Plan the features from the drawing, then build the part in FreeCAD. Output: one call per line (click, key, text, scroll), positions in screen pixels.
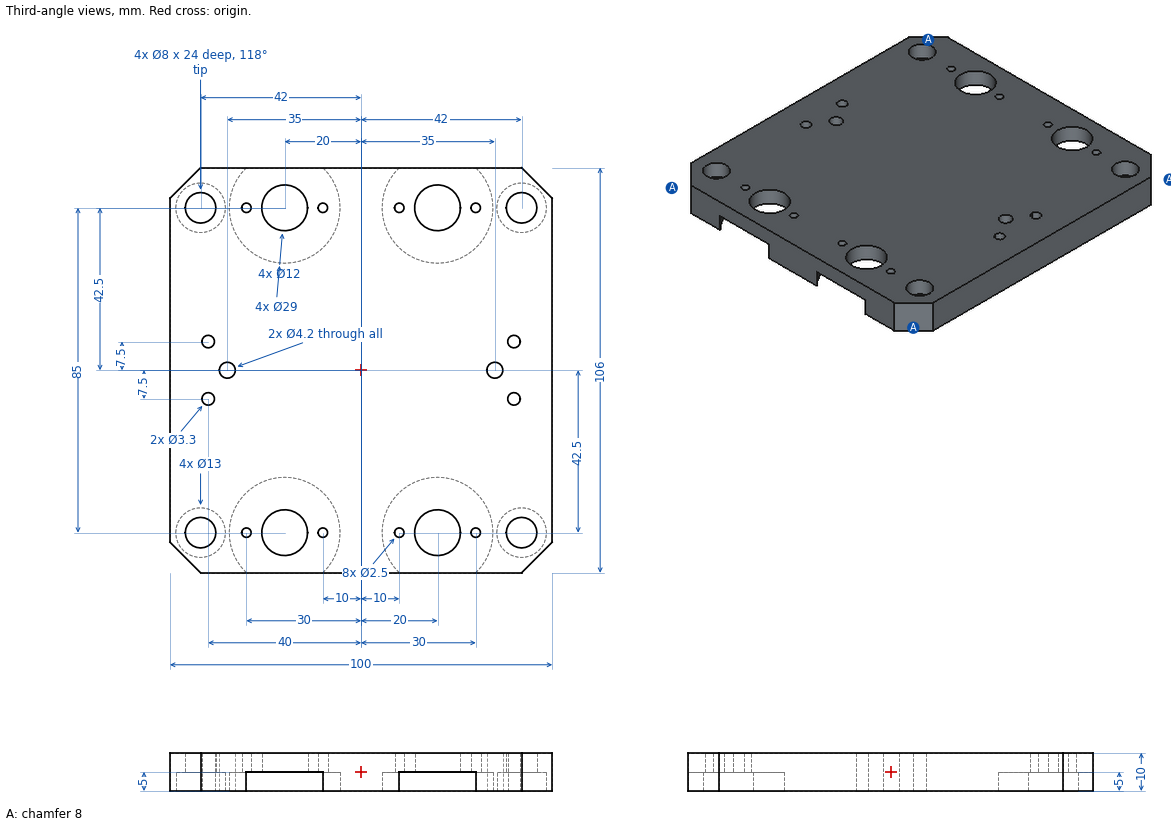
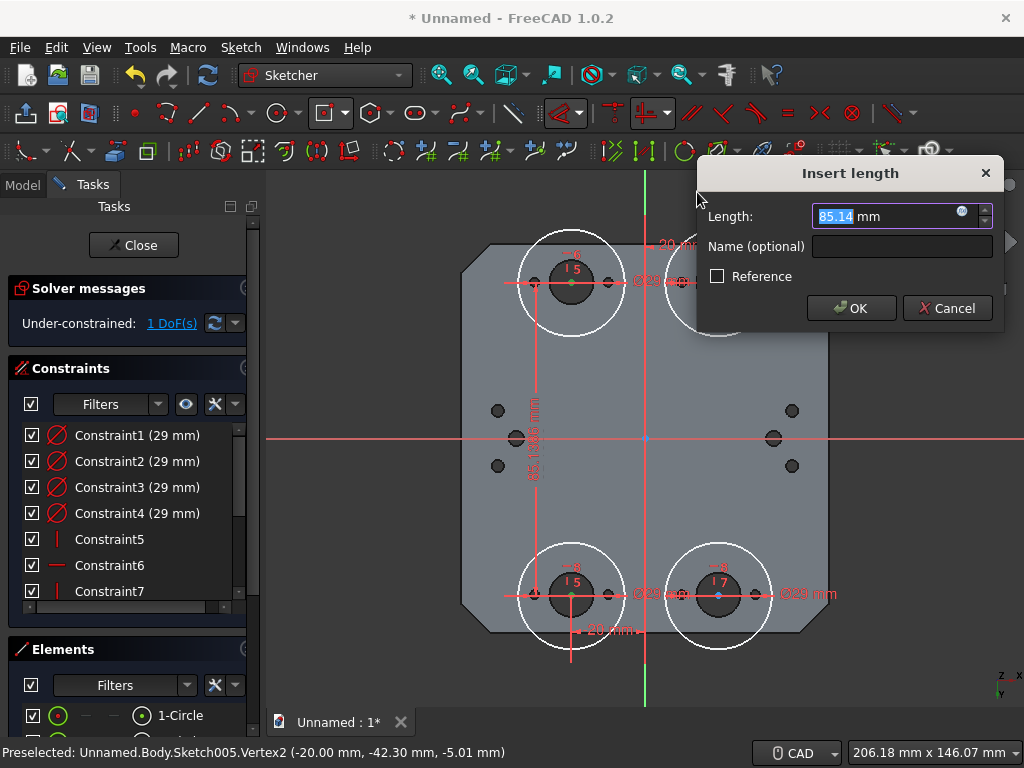
text(85)
key(Return)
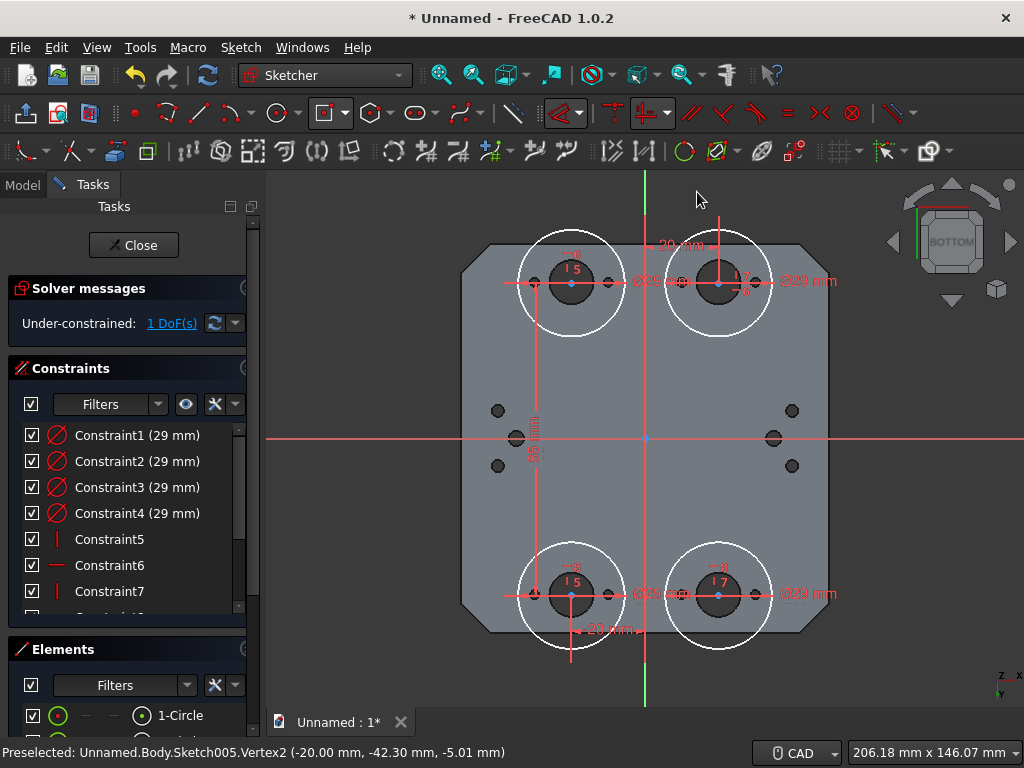
click(571, 596)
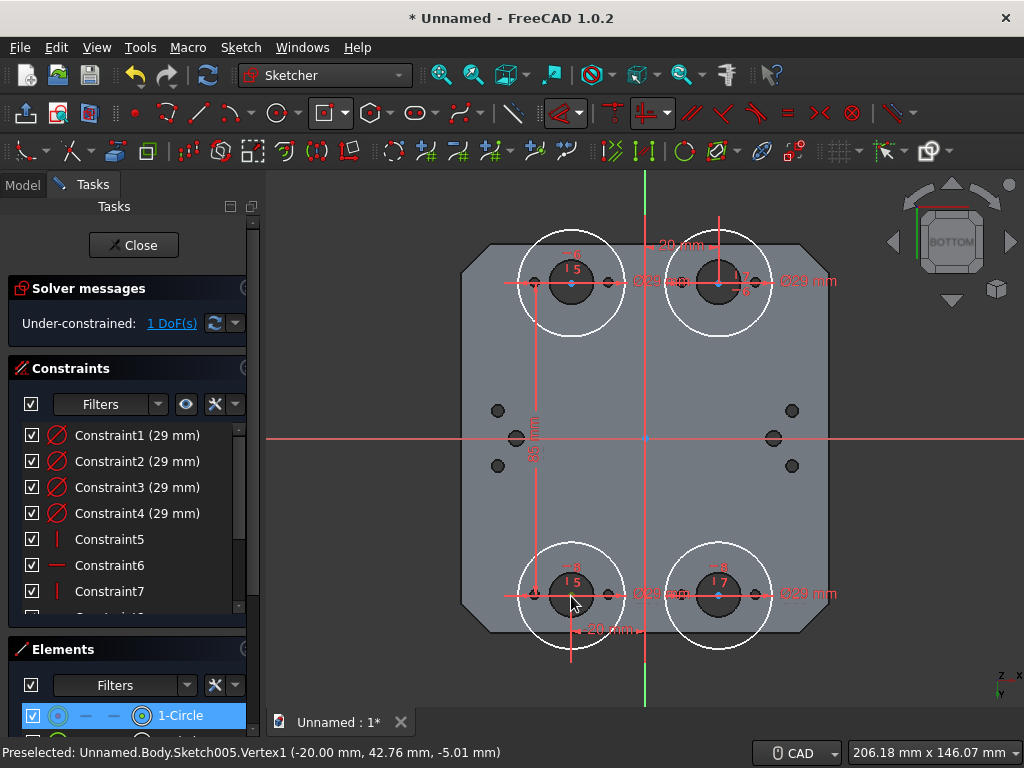
key(i)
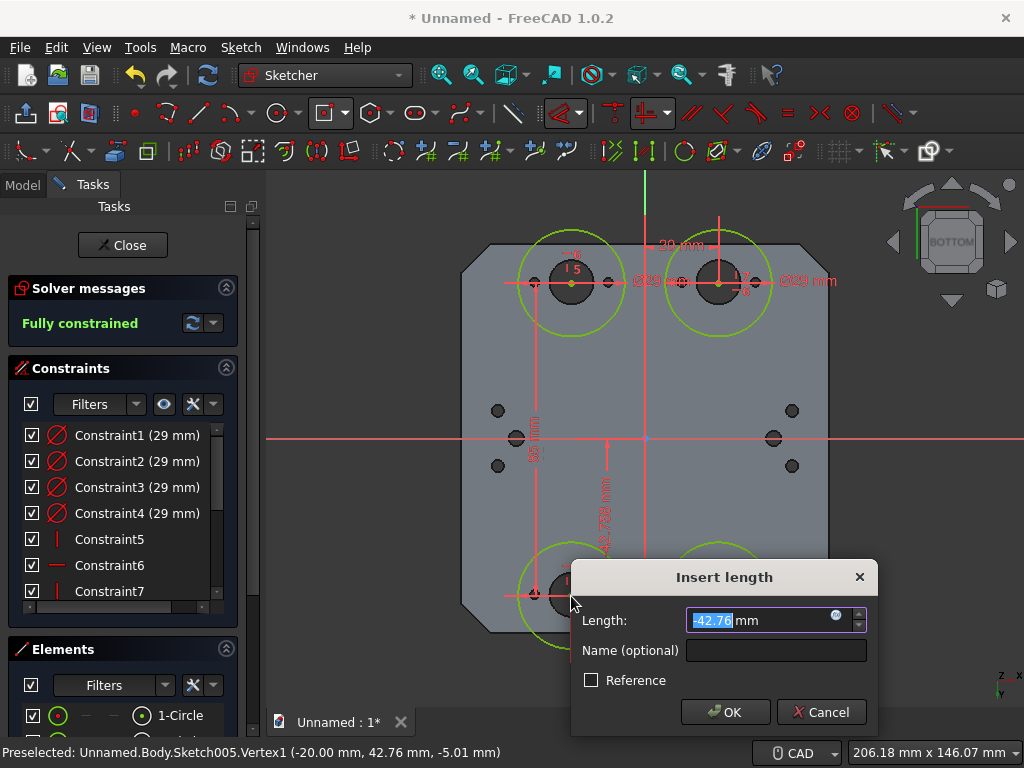
text(-42.5)
key(Return)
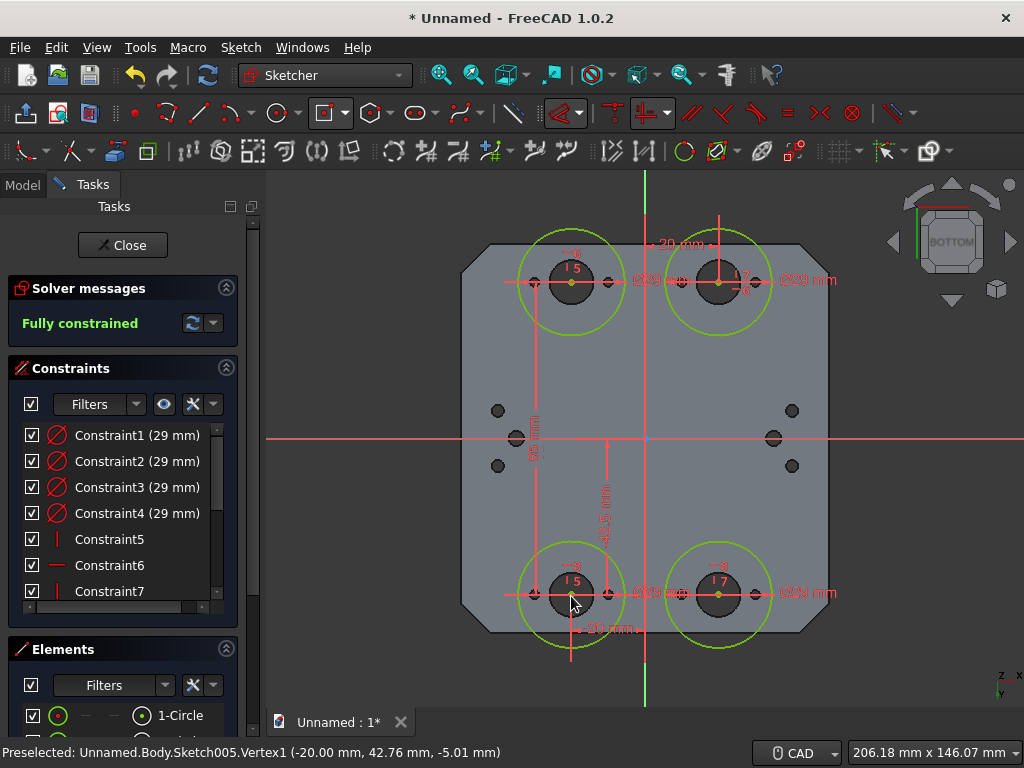
click(123, 245)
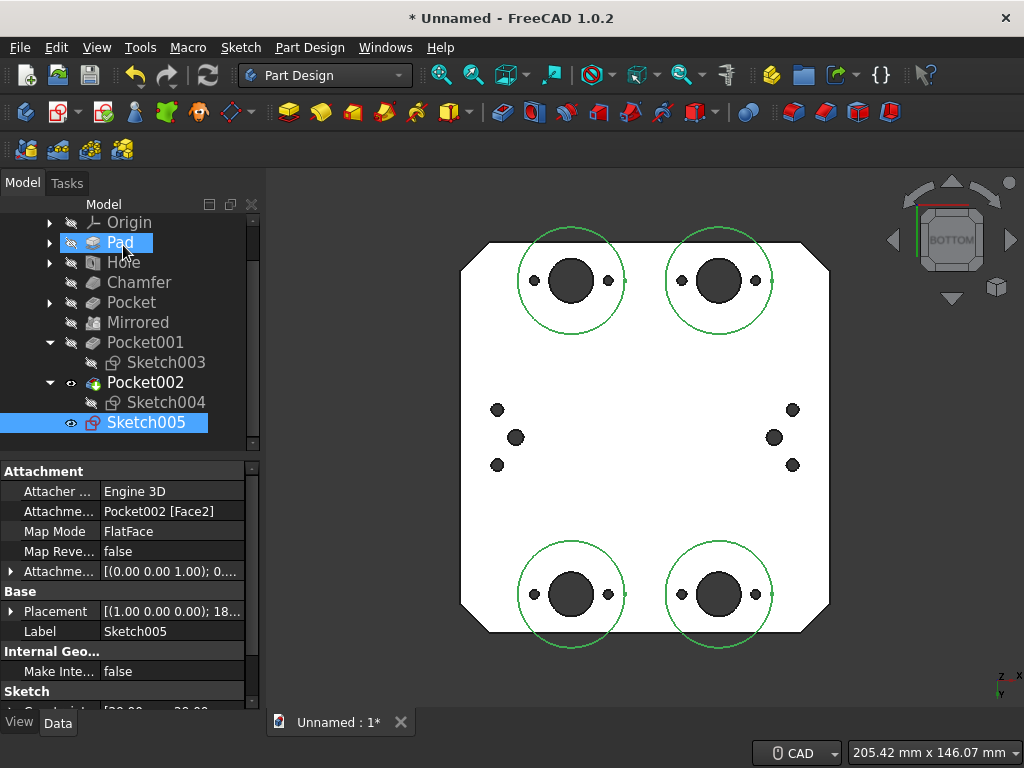
click(504, 112)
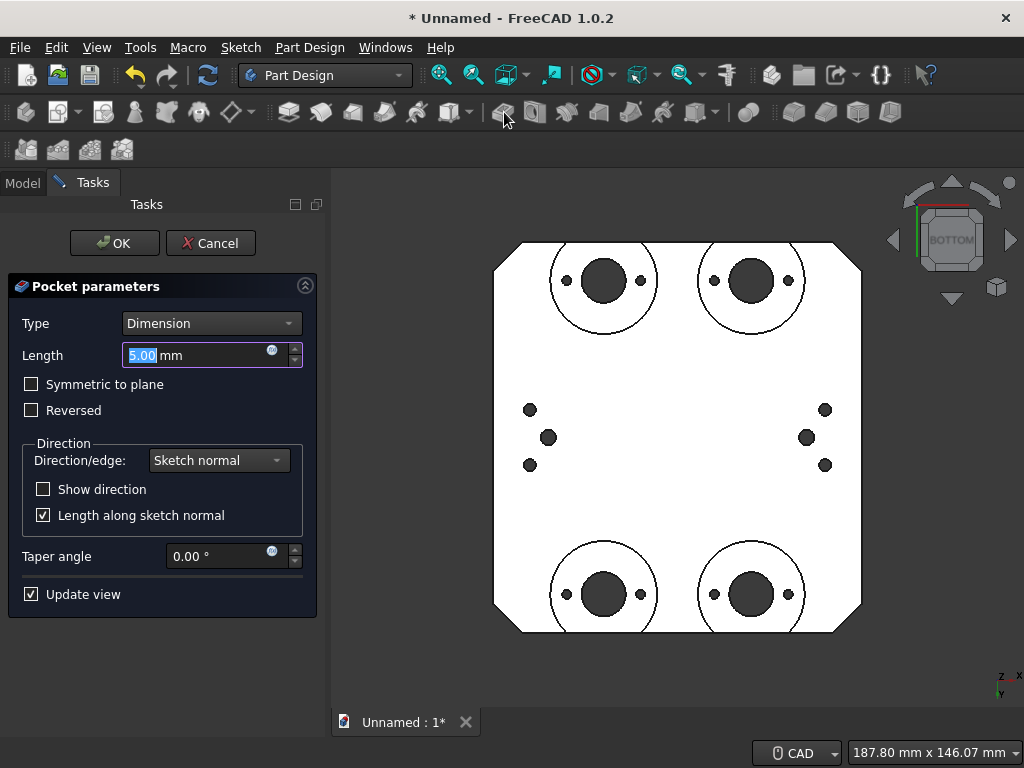
text(5)
key(Tab)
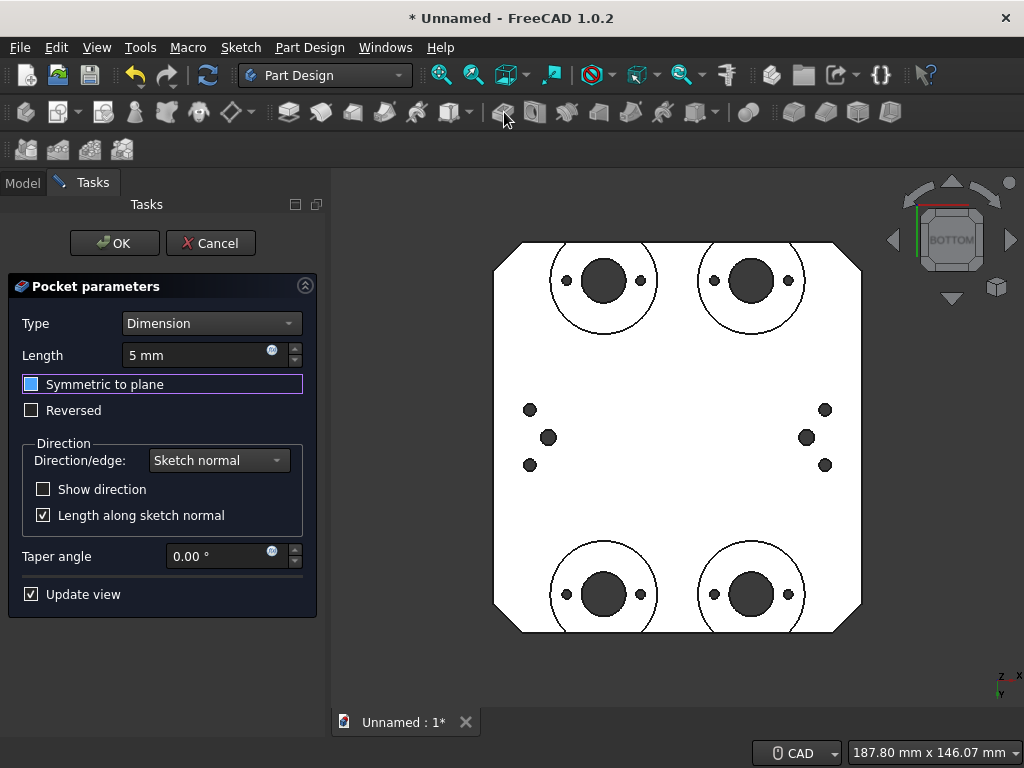
click(115, 243)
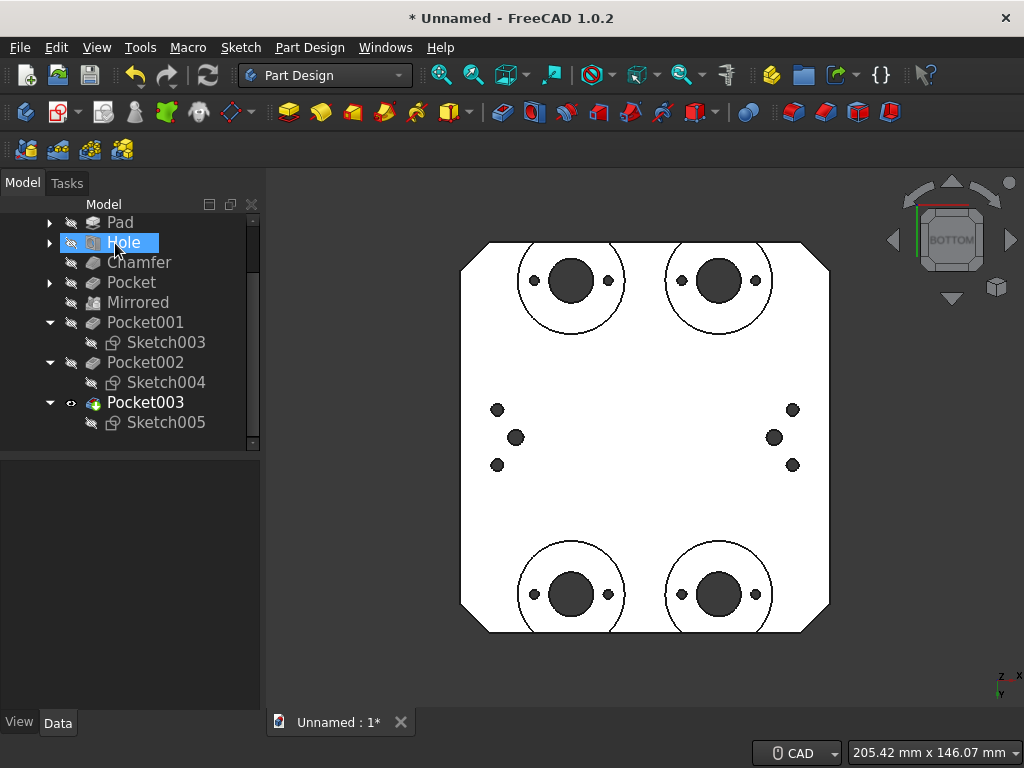
key(0)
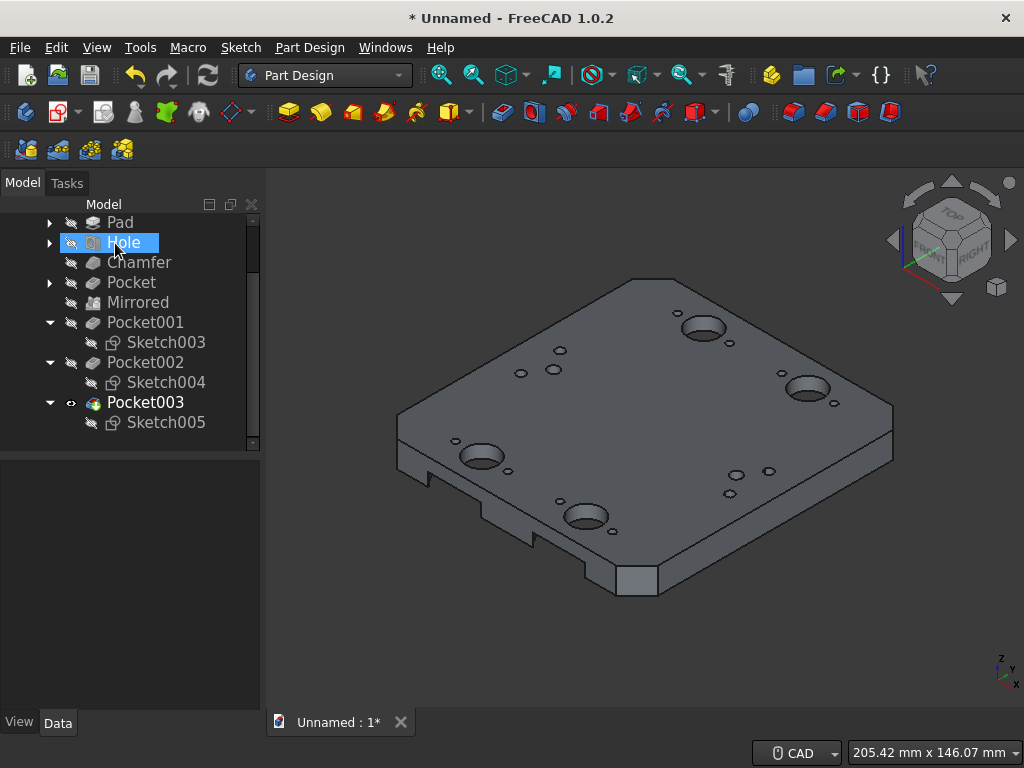
click(645, 421)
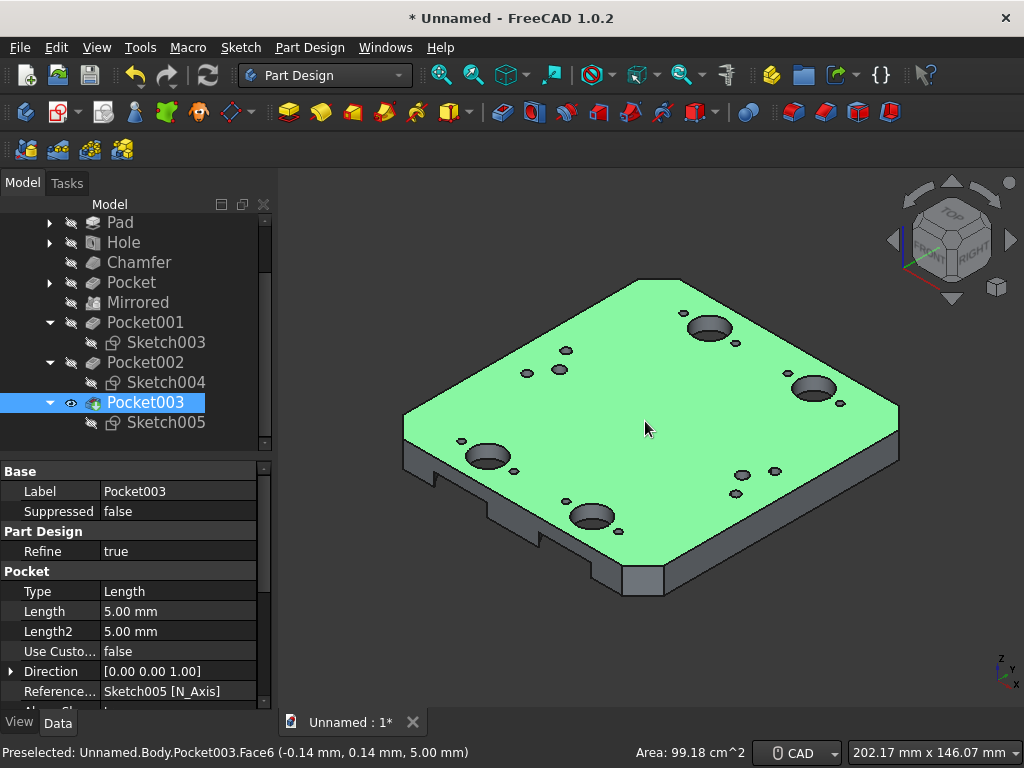
click(58, 112)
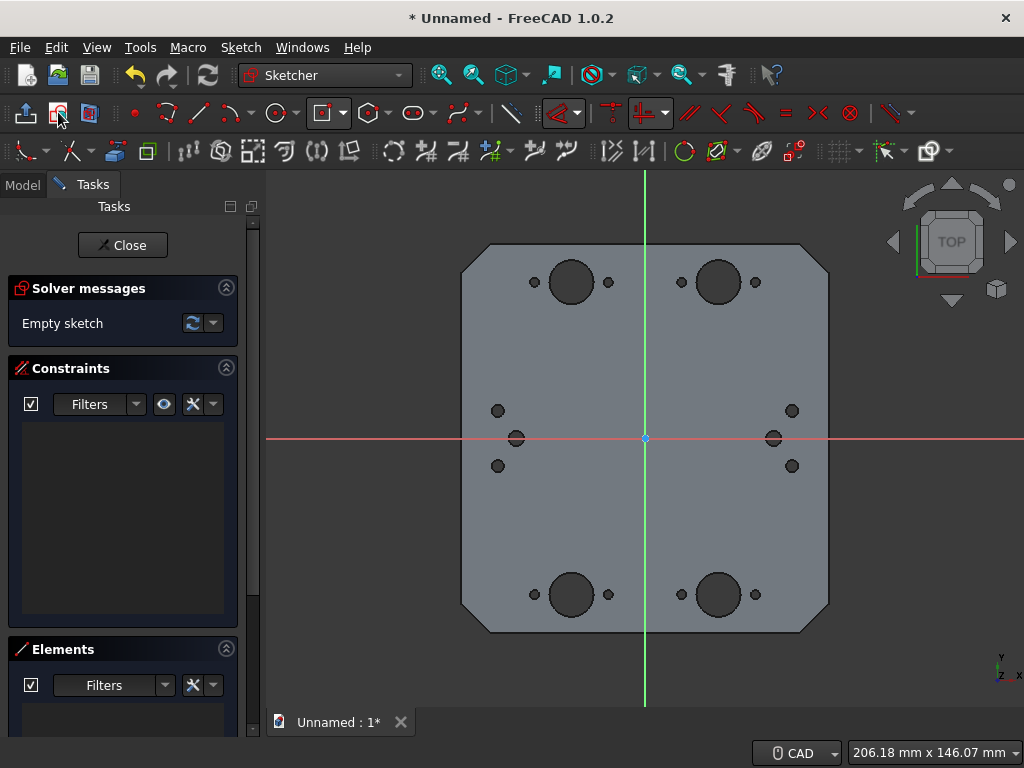
click(276, 114)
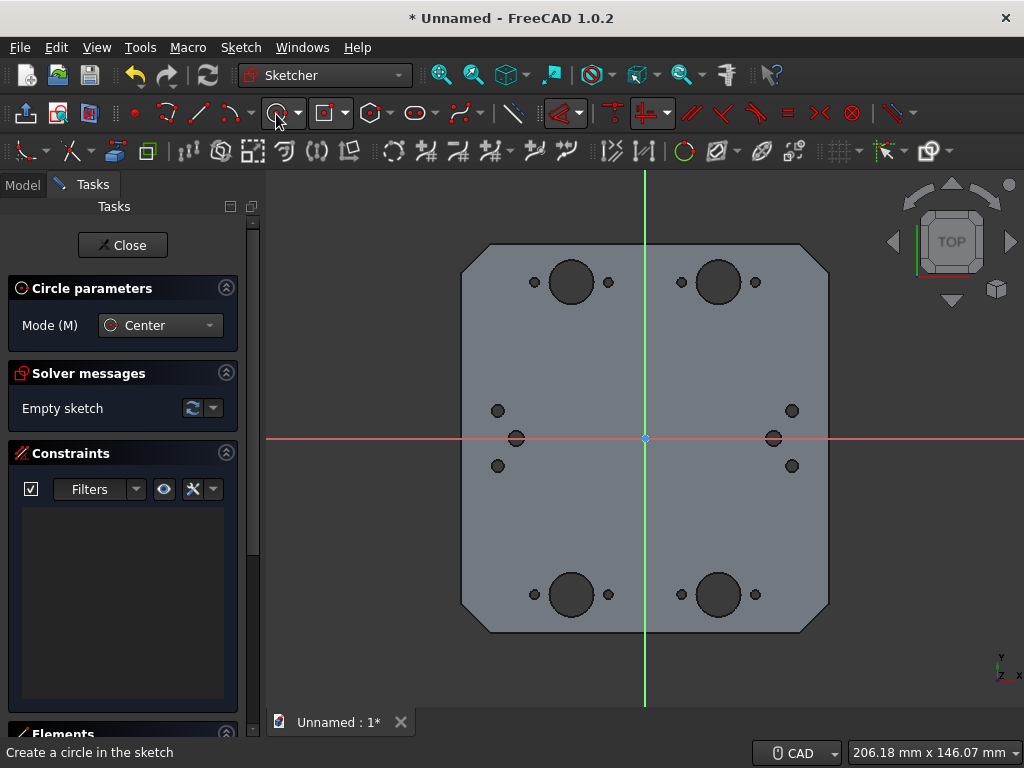
scroll(491, 282, up, 3)